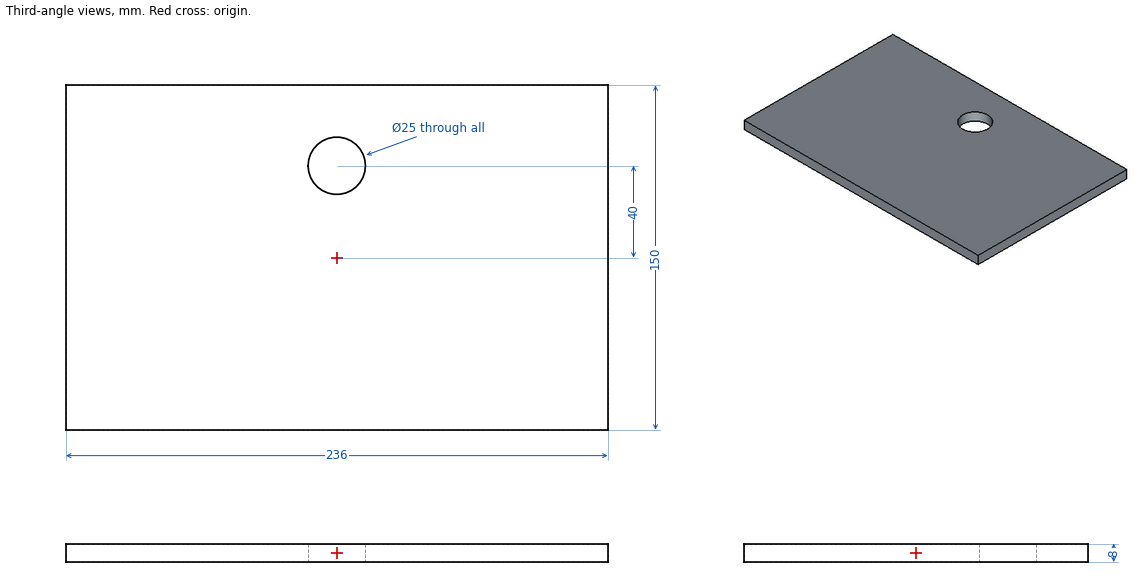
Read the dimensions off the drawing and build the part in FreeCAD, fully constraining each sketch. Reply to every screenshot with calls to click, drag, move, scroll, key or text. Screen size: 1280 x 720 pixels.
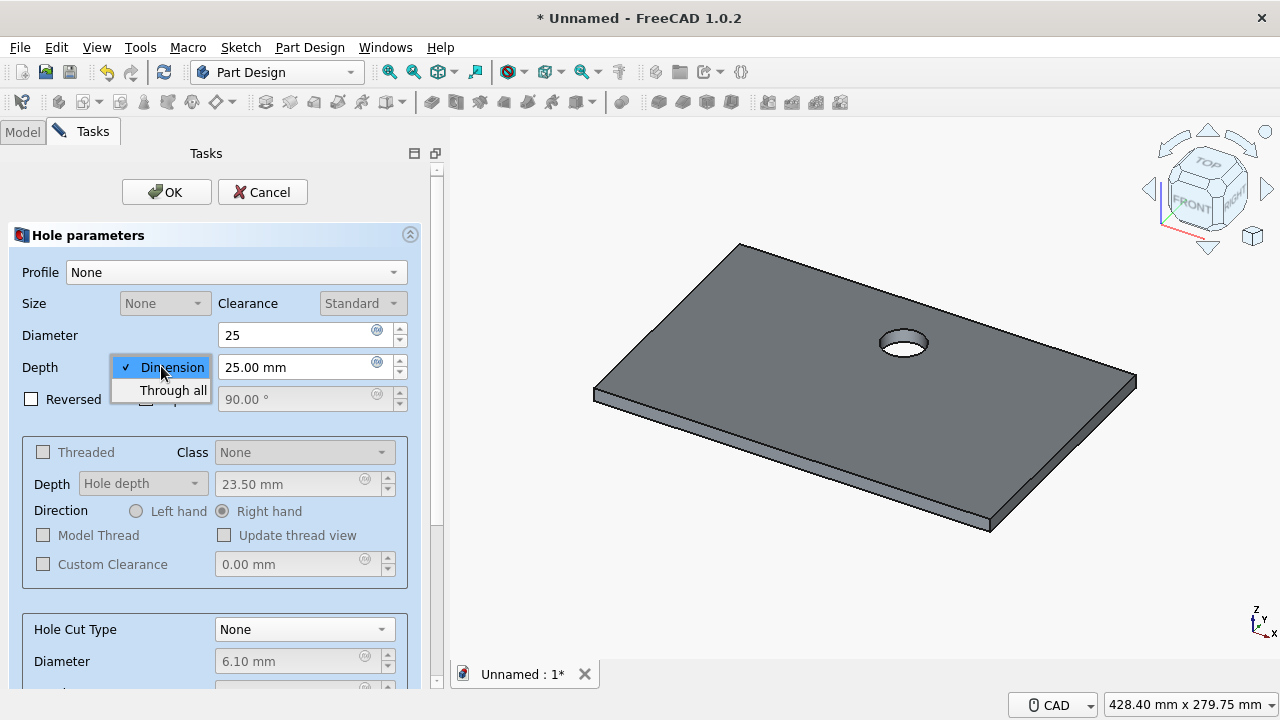
click(160, 390)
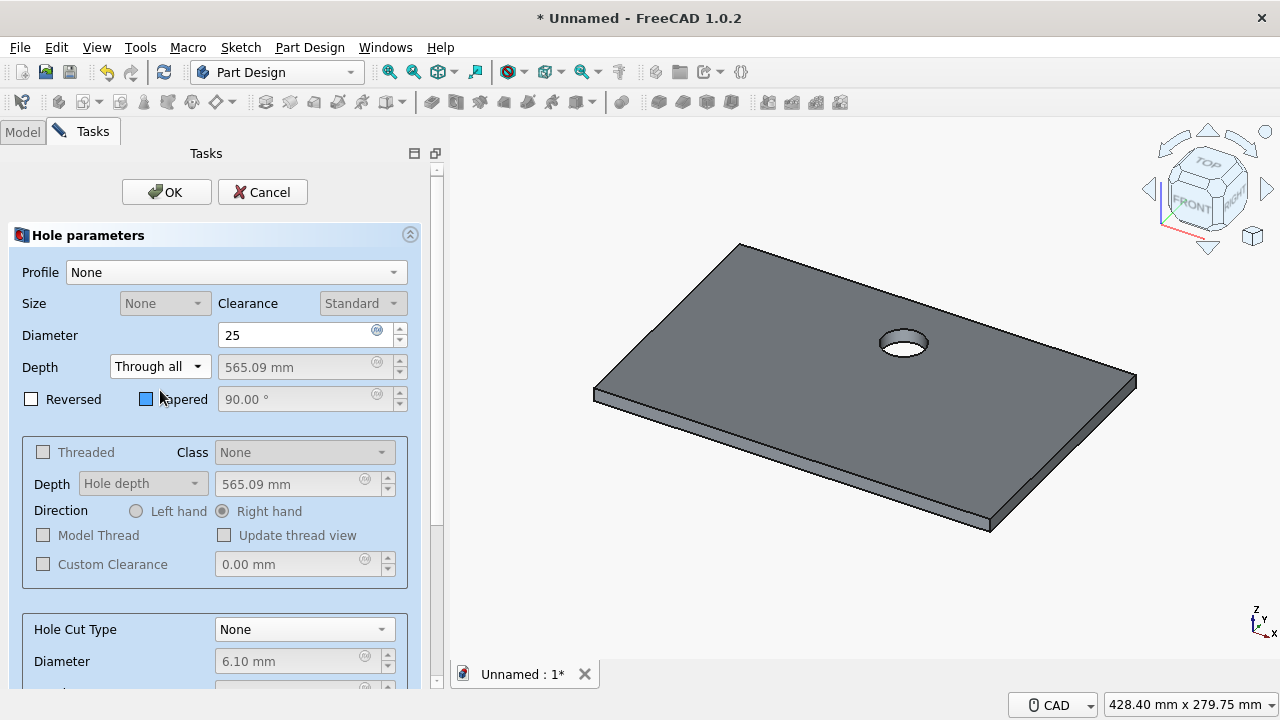
click(167, 192)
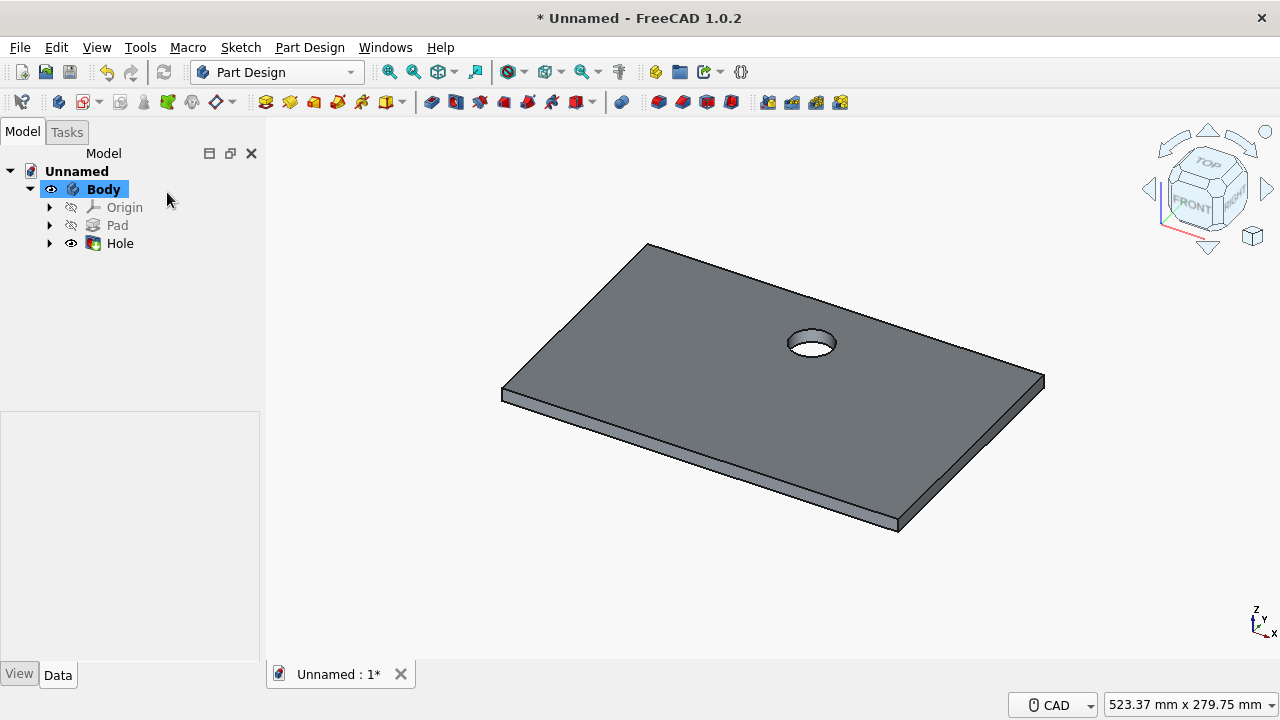
key(0)